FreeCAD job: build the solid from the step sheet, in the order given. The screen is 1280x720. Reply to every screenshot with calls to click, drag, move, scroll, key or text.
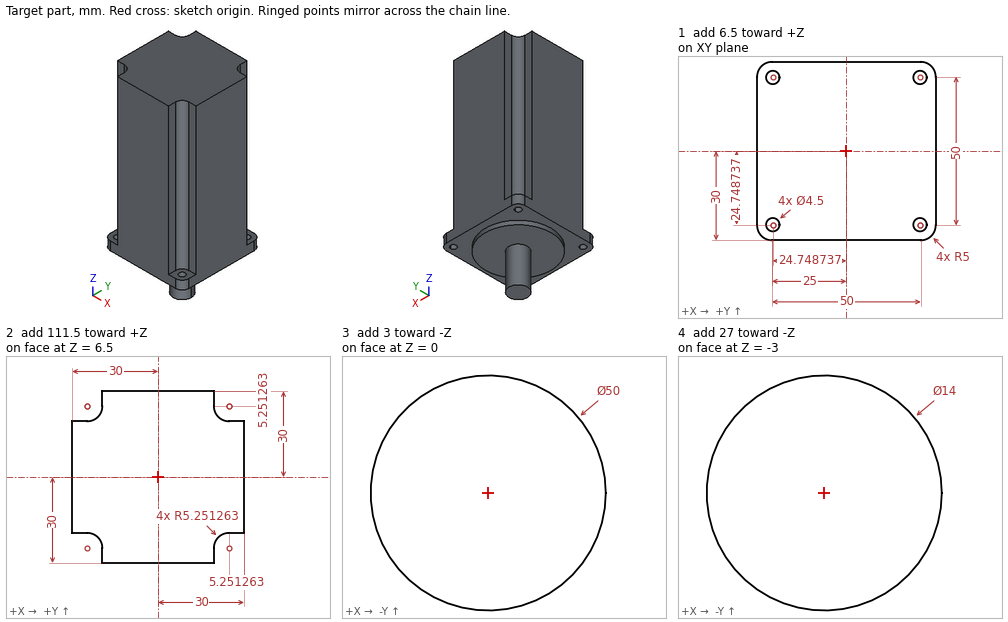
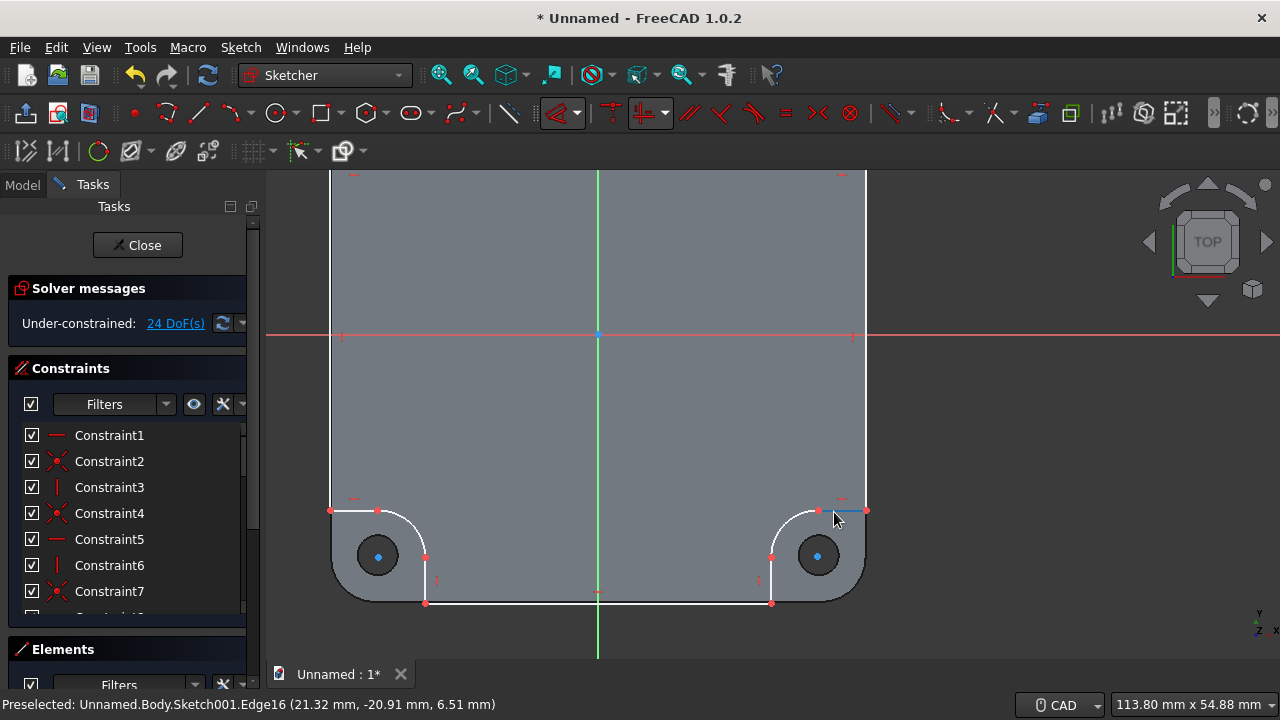
click(833, 511)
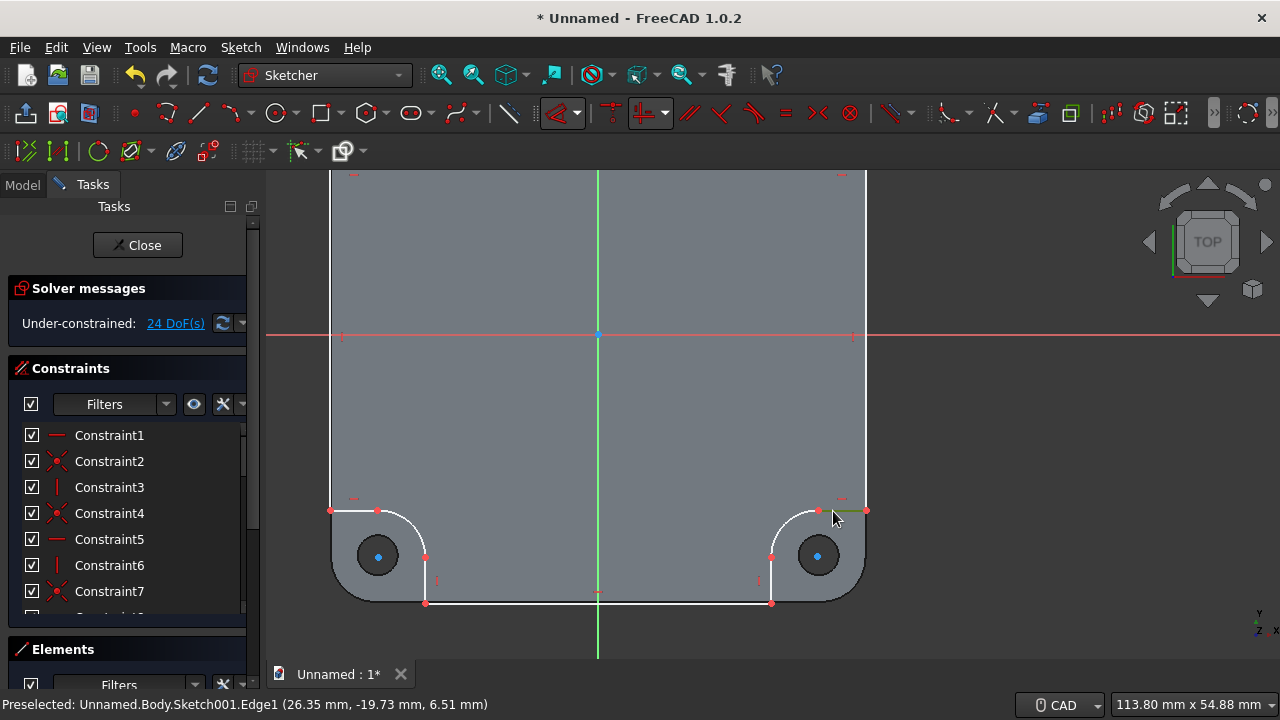
click(797, 515)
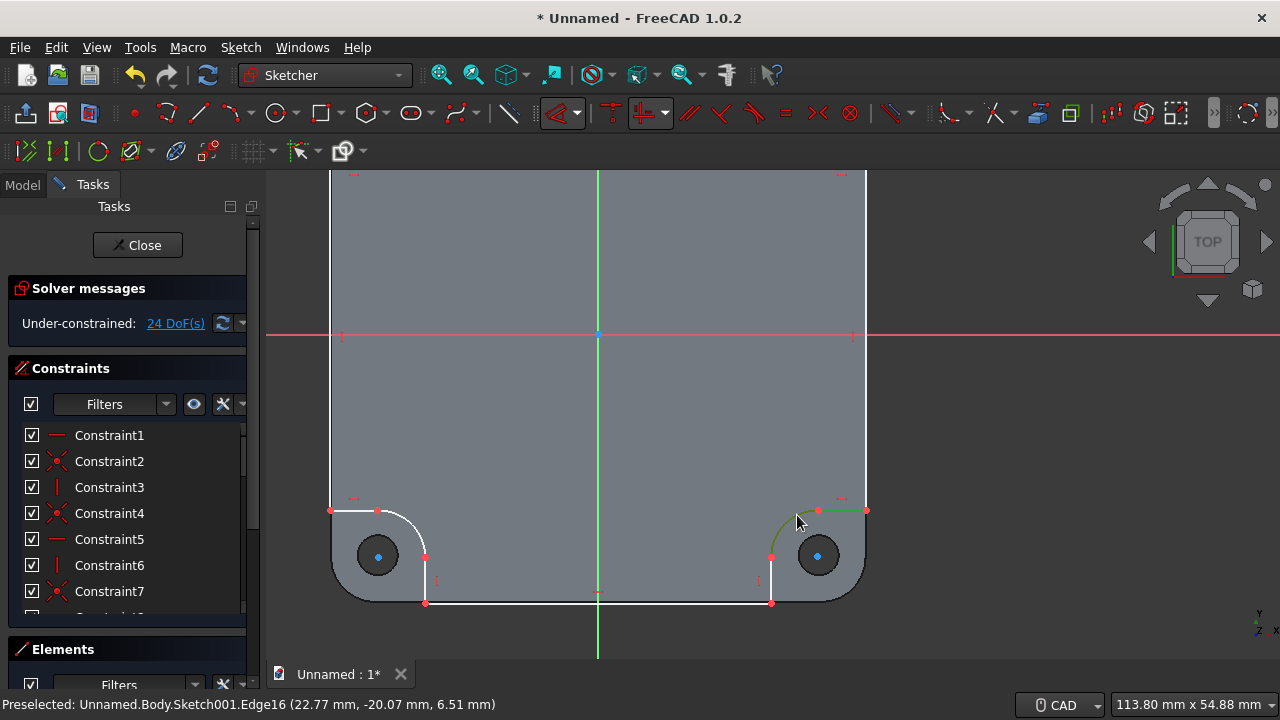
key(t)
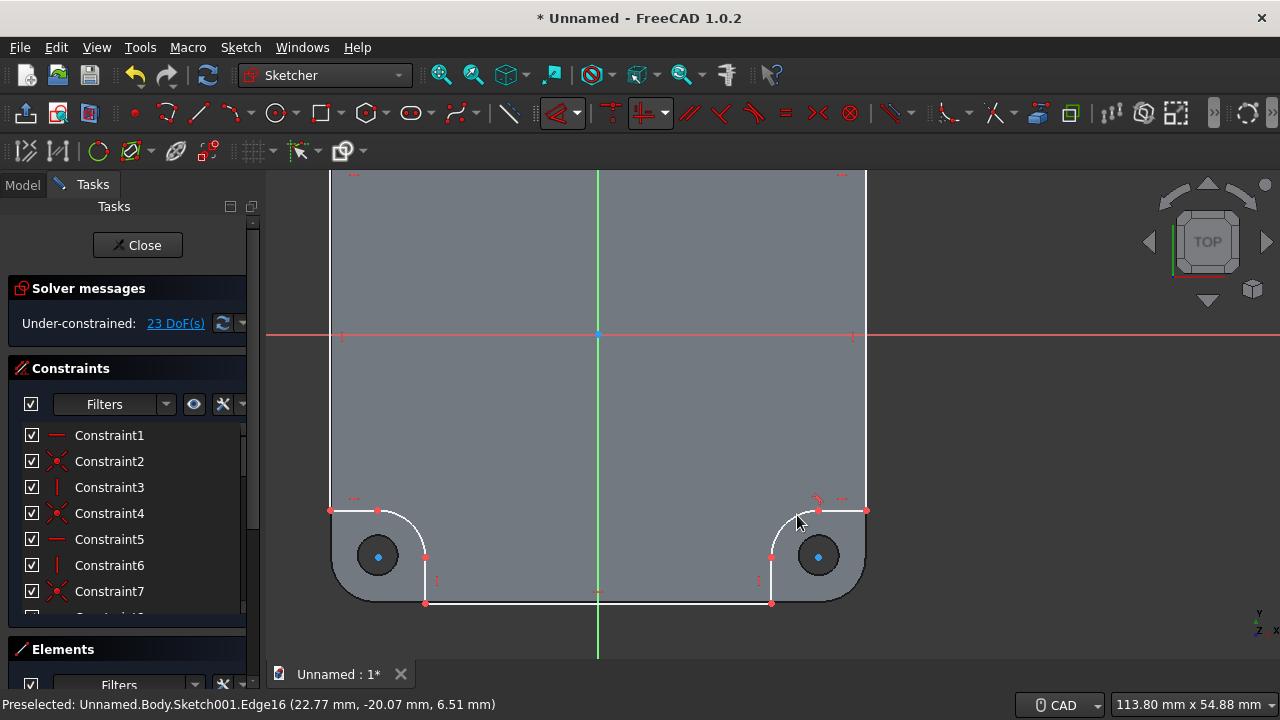
scroll(834, 511, down, 3)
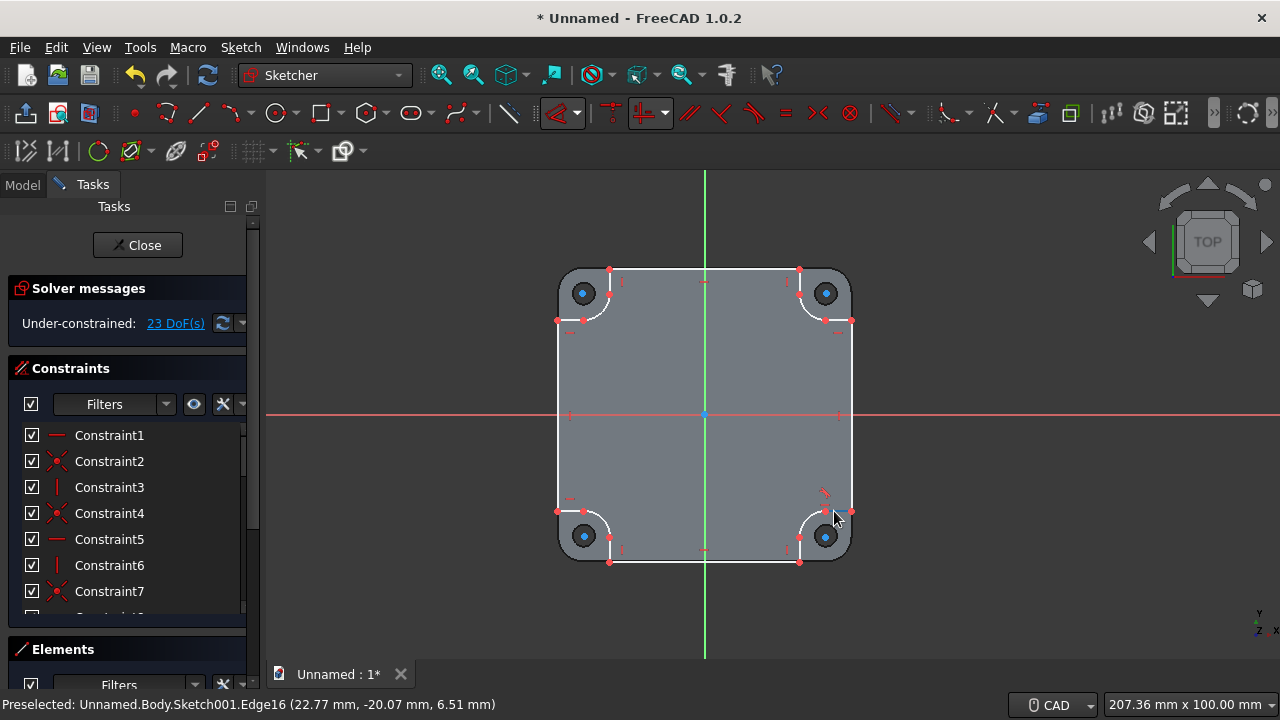
scroll(844, 320, up, 3)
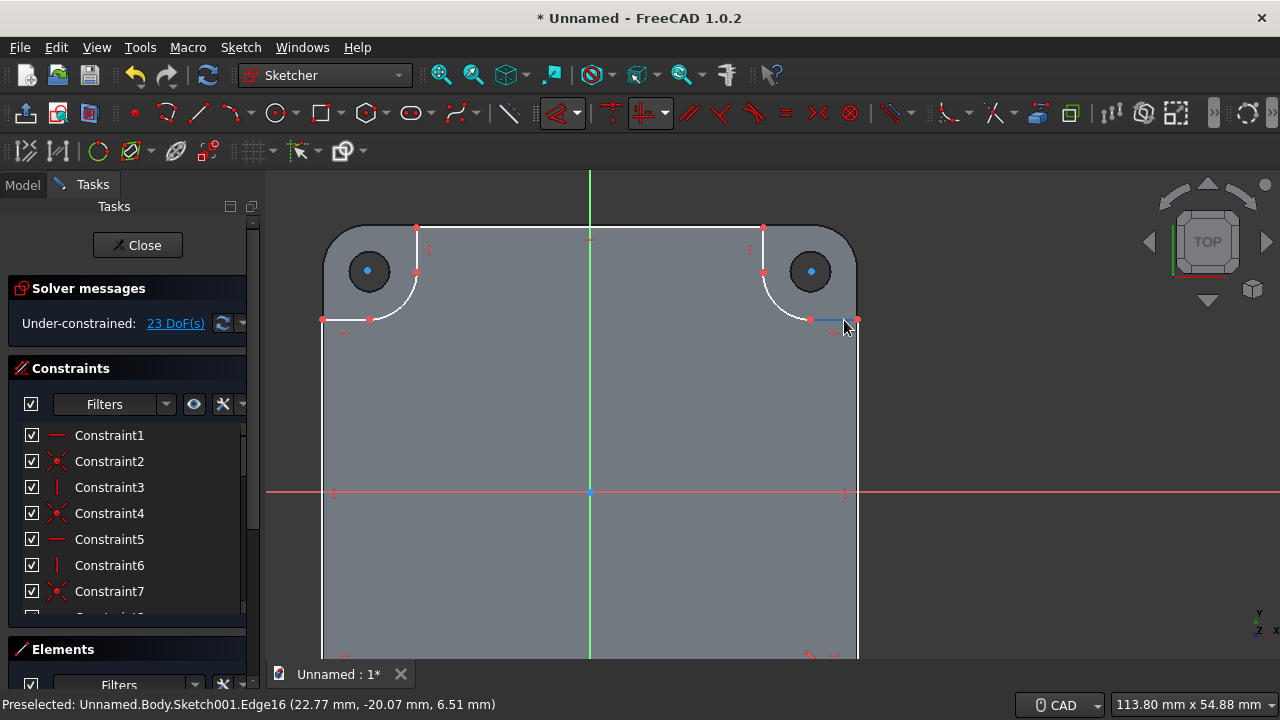
click(844, 320)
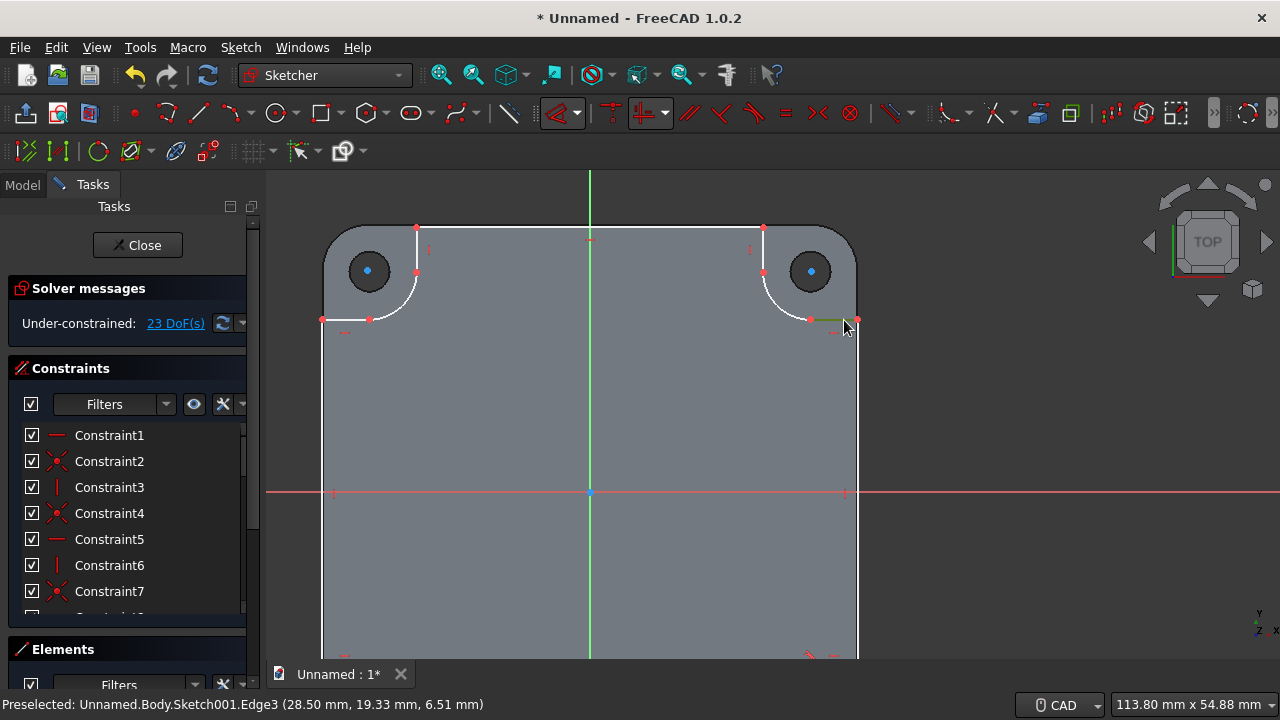
click(769, 294)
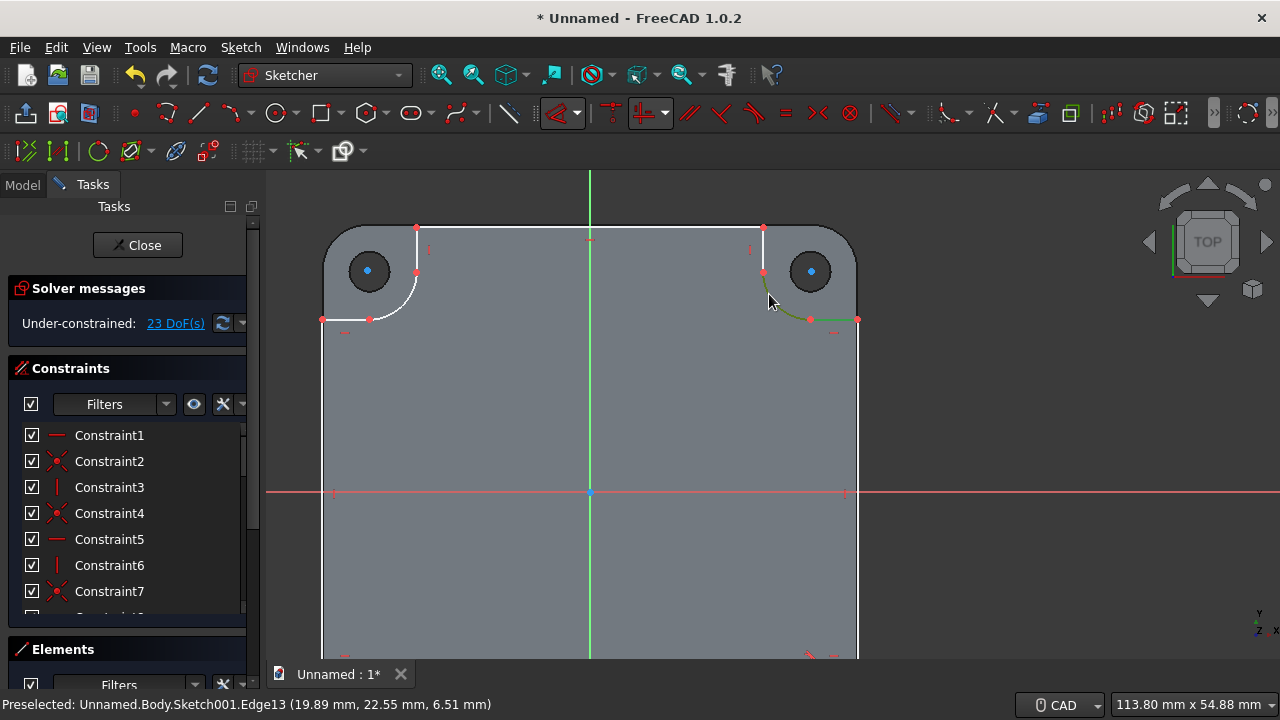
key(t)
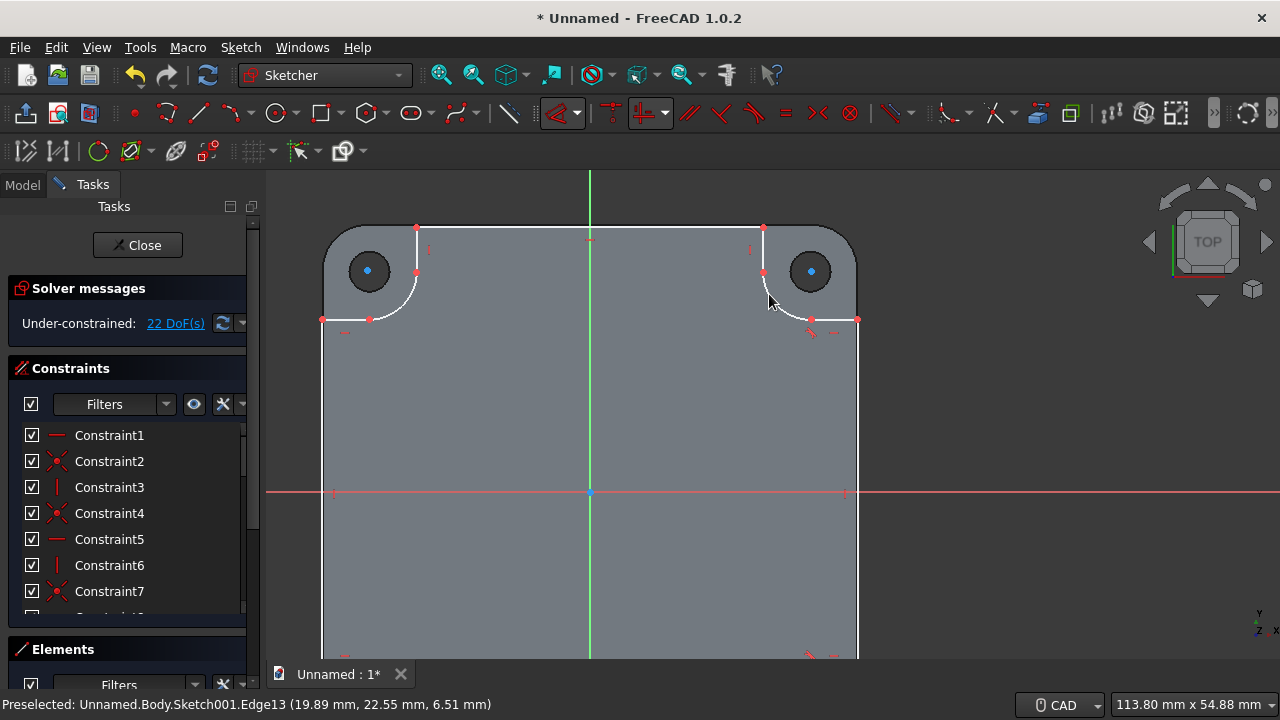
click(763, 259)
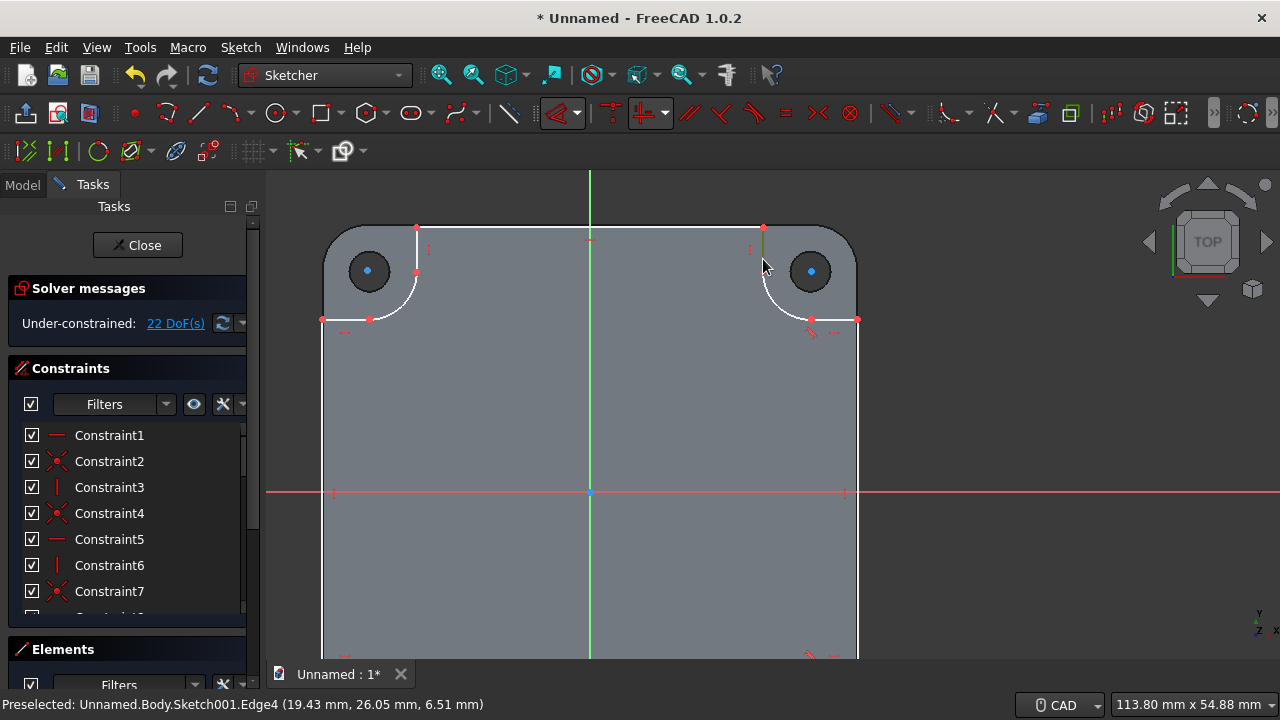
click(769, 294)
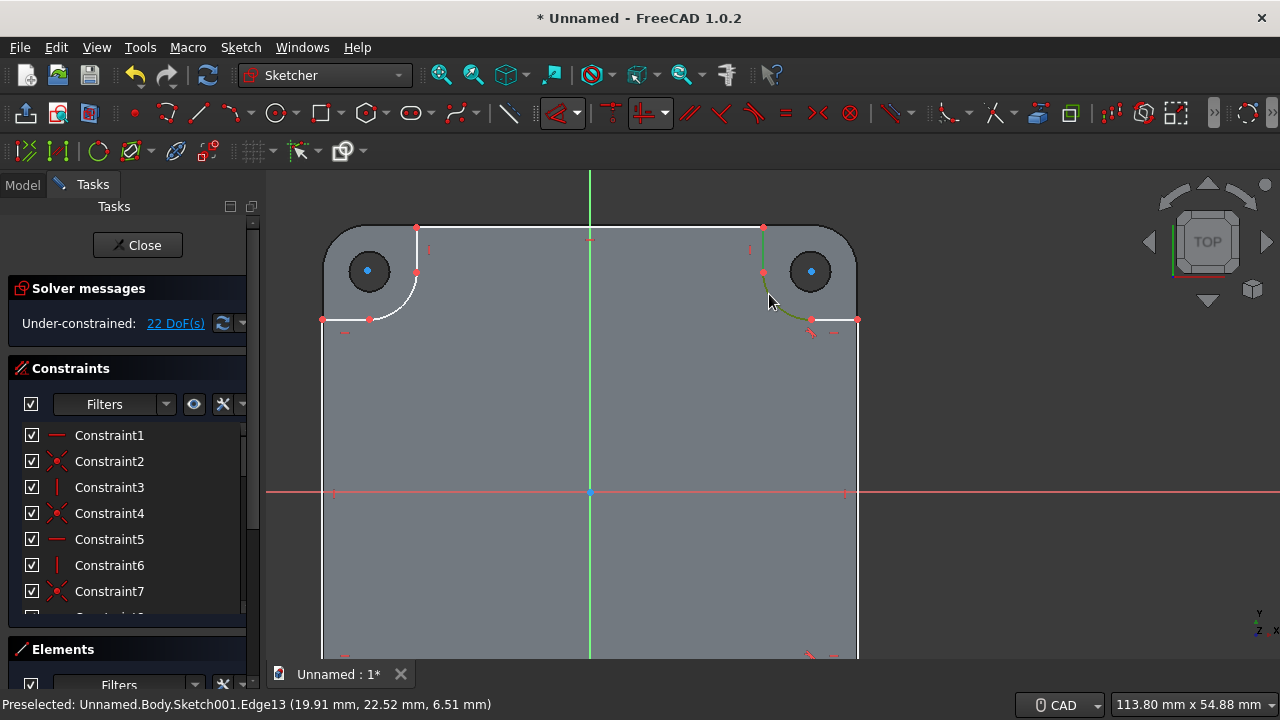
key(t)